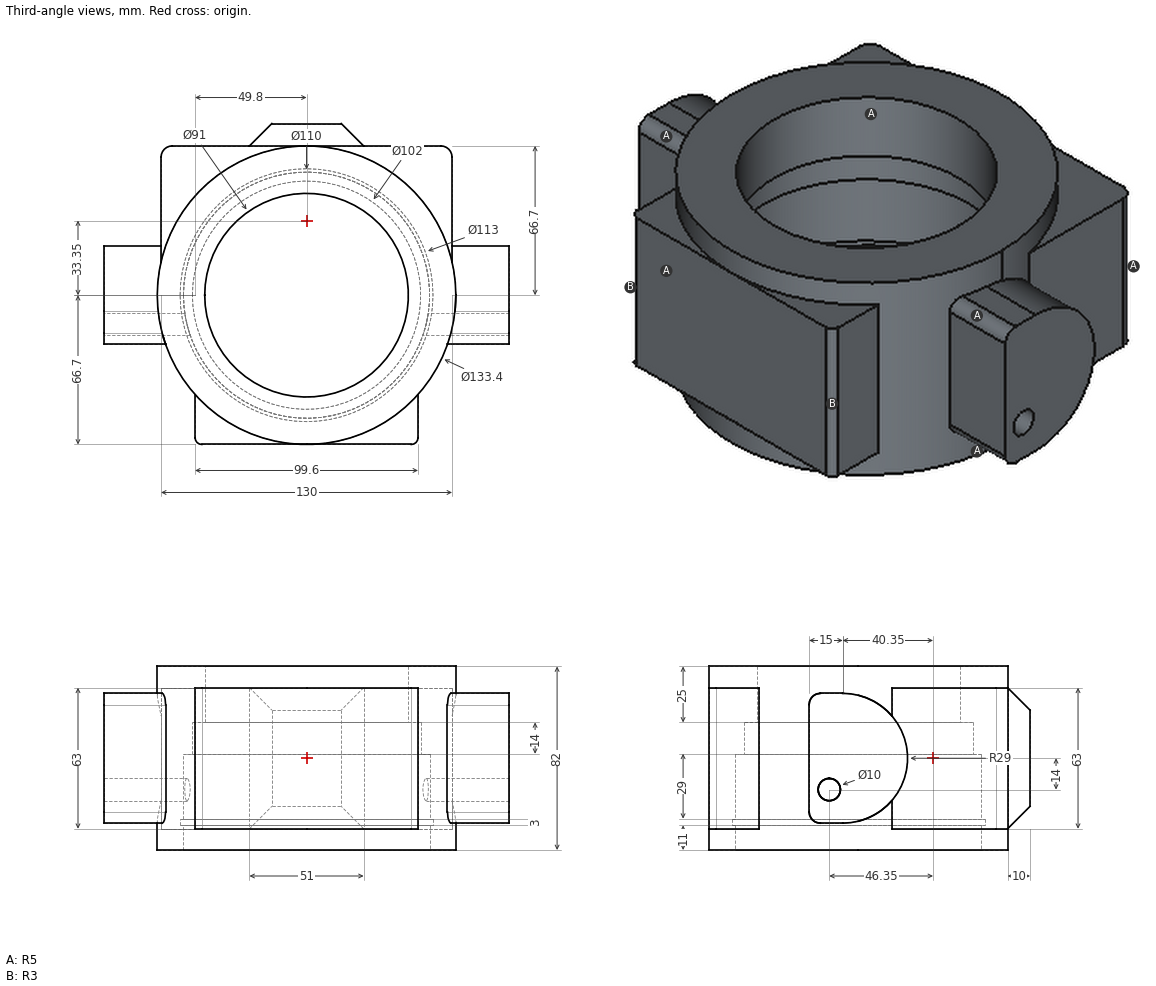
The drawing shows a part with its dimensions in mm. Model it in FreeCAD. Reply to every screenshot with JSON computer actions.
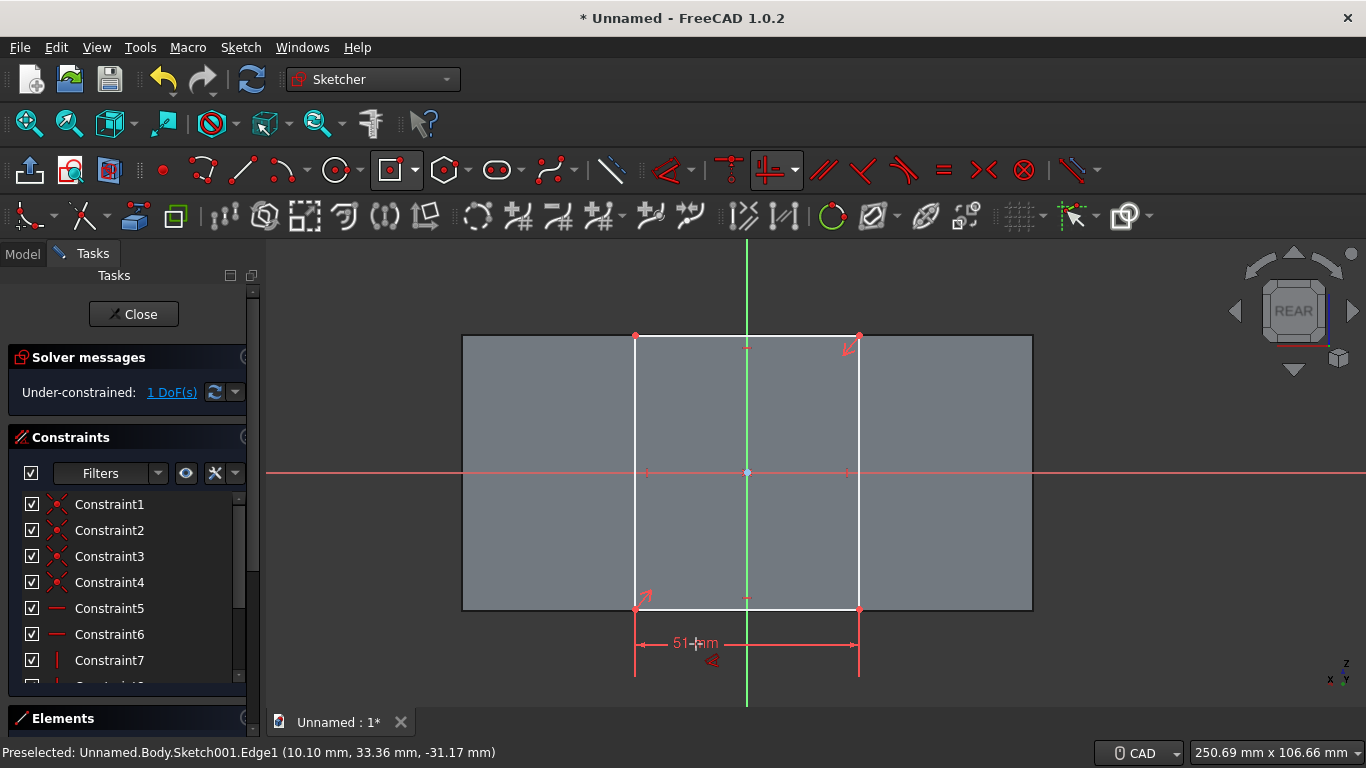
{"action": "left_click", "coordinate": [859, 527]}
{"action": "left_click", "coordinate": [893, 410]}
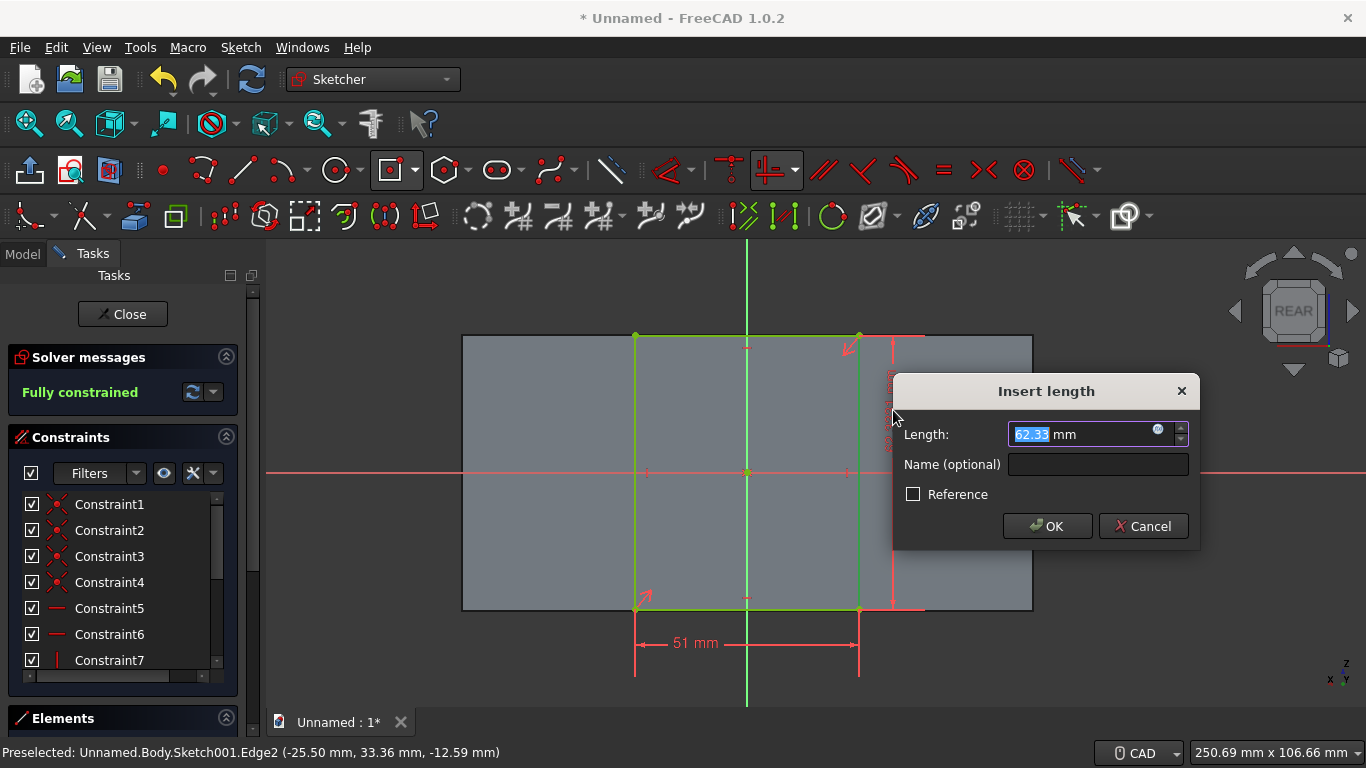
{"action": "type", "text": "63"}
{"action": "key", "text": "Return"}
{"action": "key", "text": "Escape"}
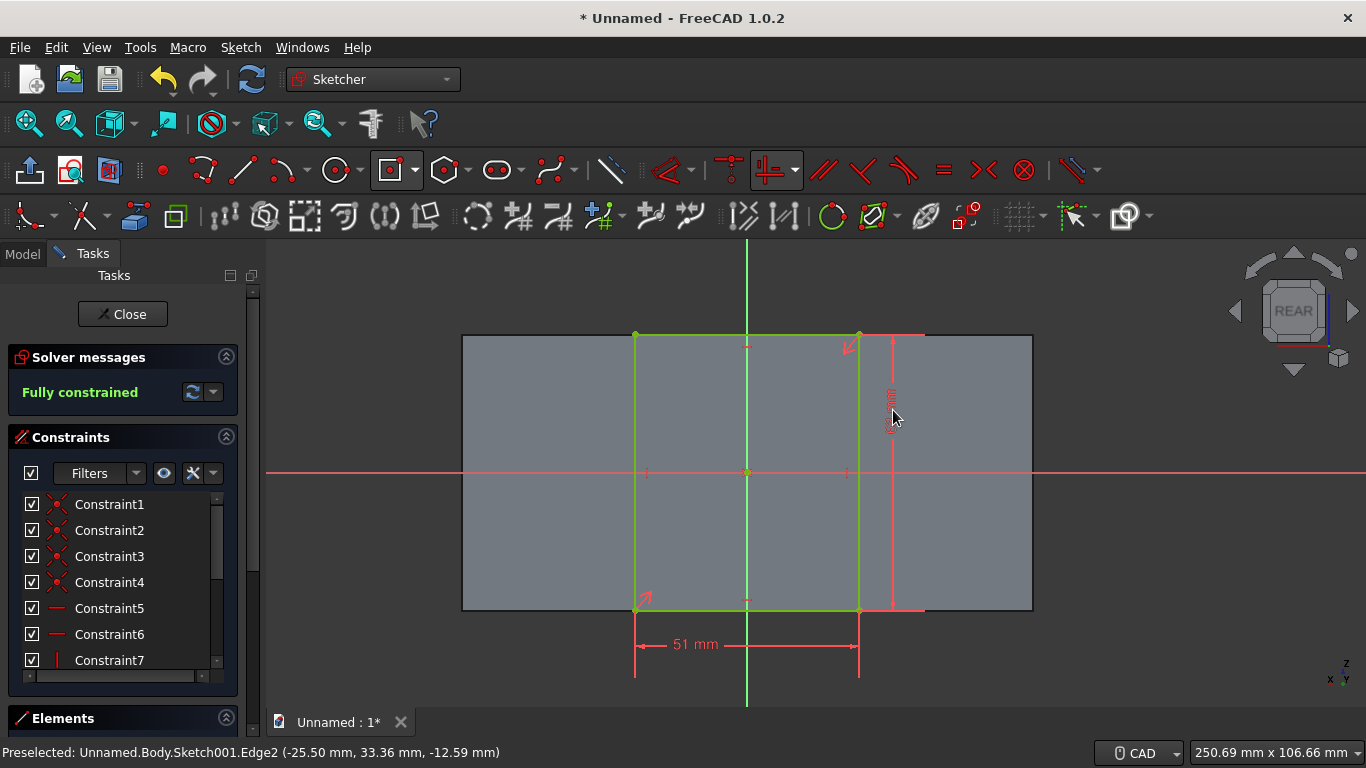
{"action": "left_click", "coordinate": [123, 314]}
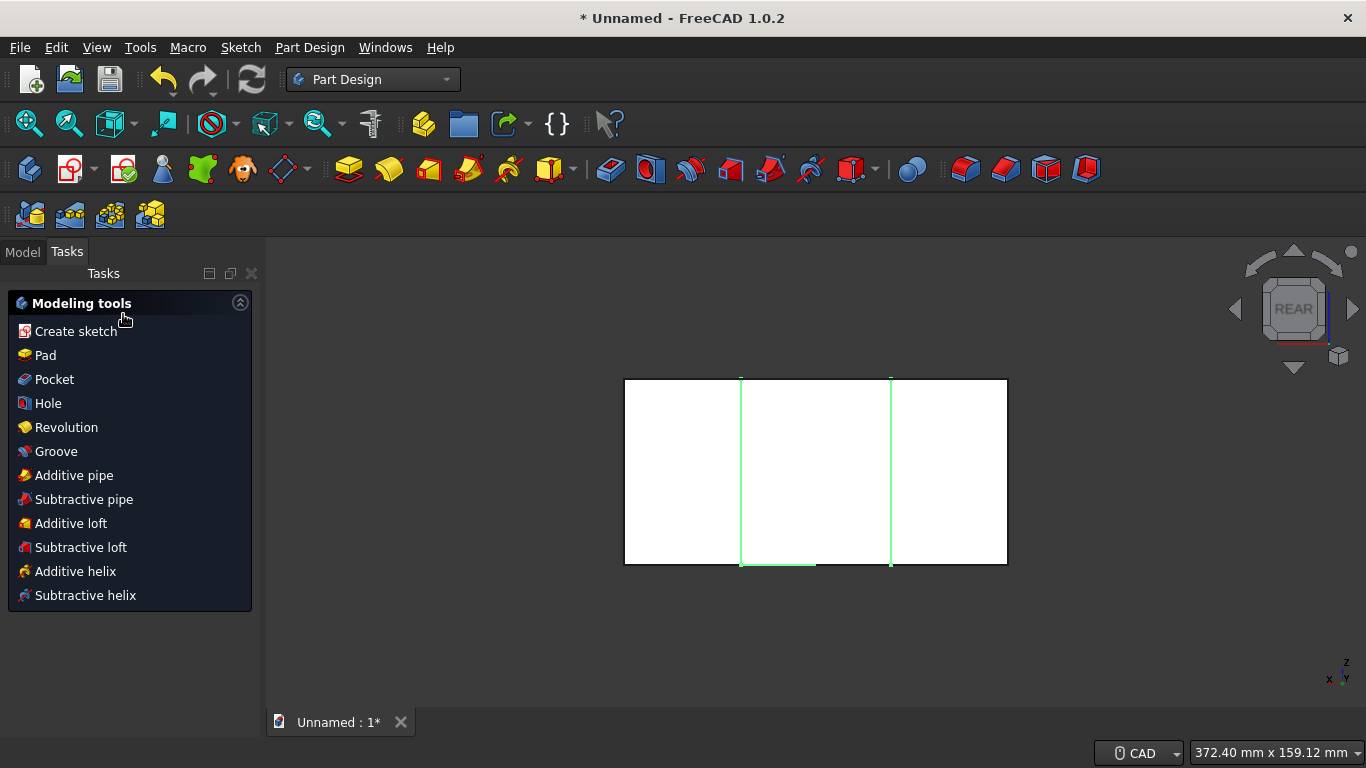
{"action": "left_click", "coordinate": [350, 170]}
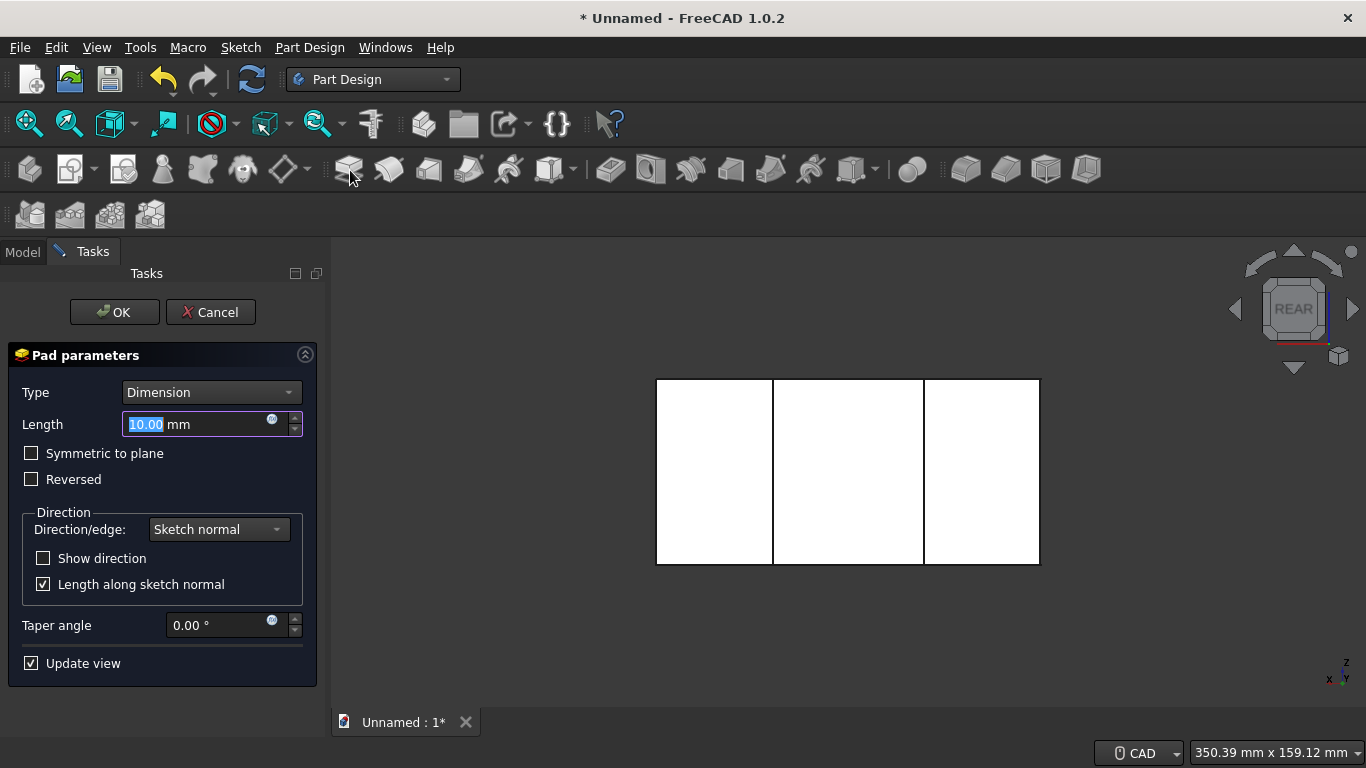
{"action": "type", "text": "10"}
{"action": "key", "text": "Tab"}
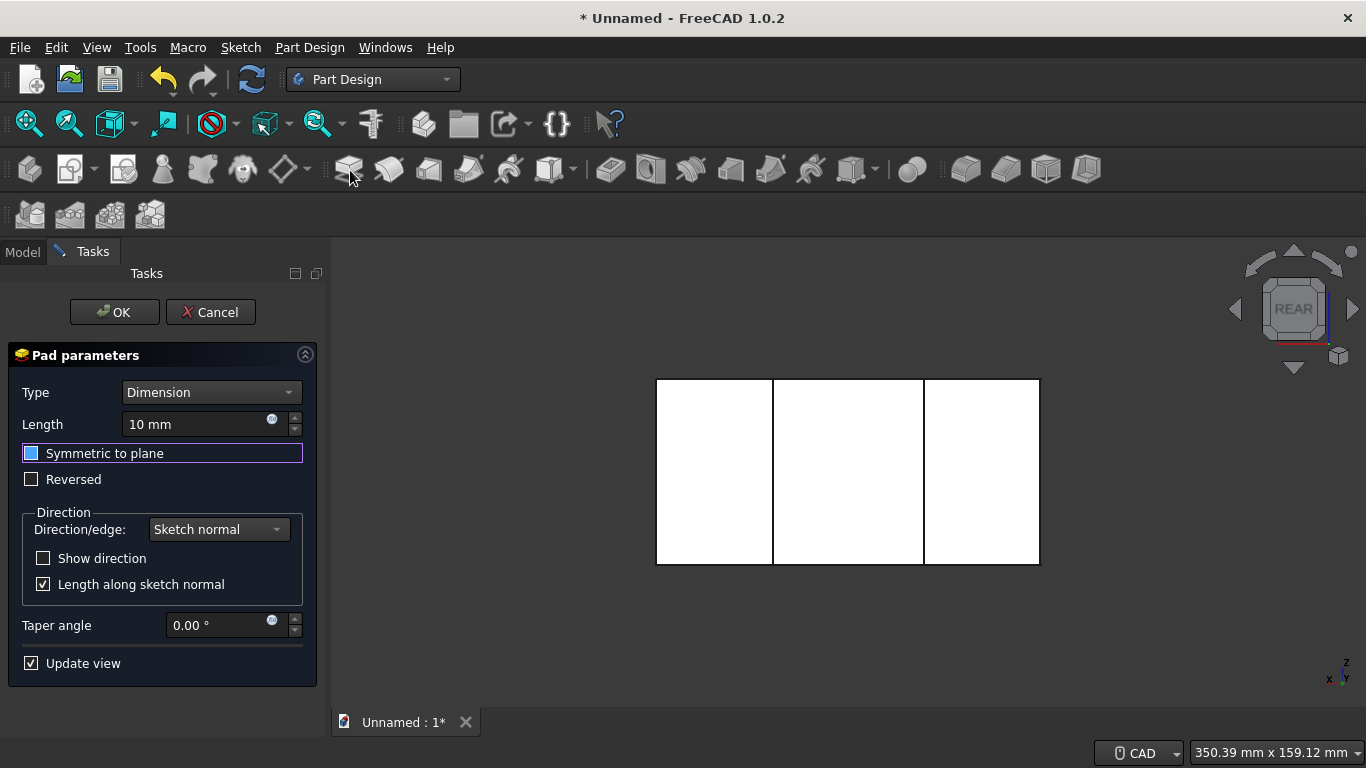
{"action": "triple_click", "coordinate": [226, 625]}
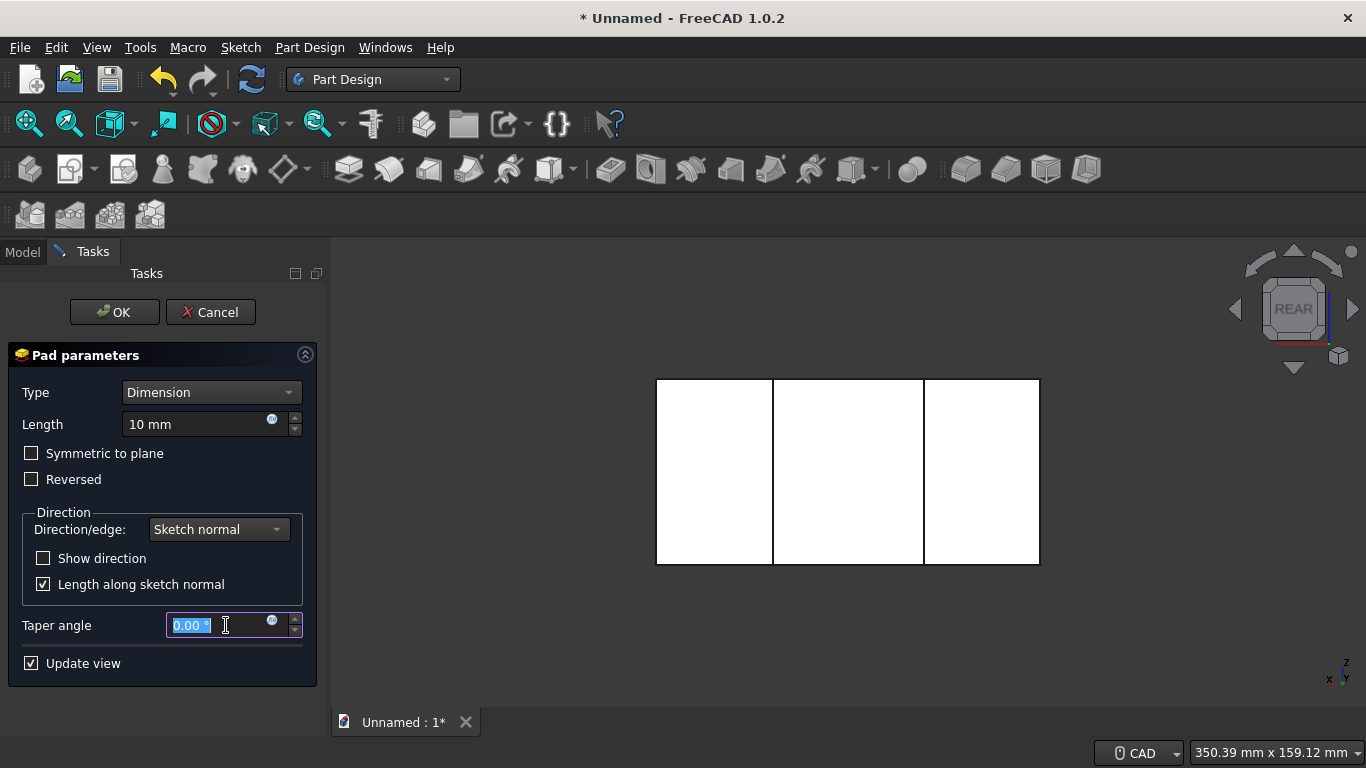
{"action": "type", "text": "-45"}
{"action": "key", "text": "Tab"}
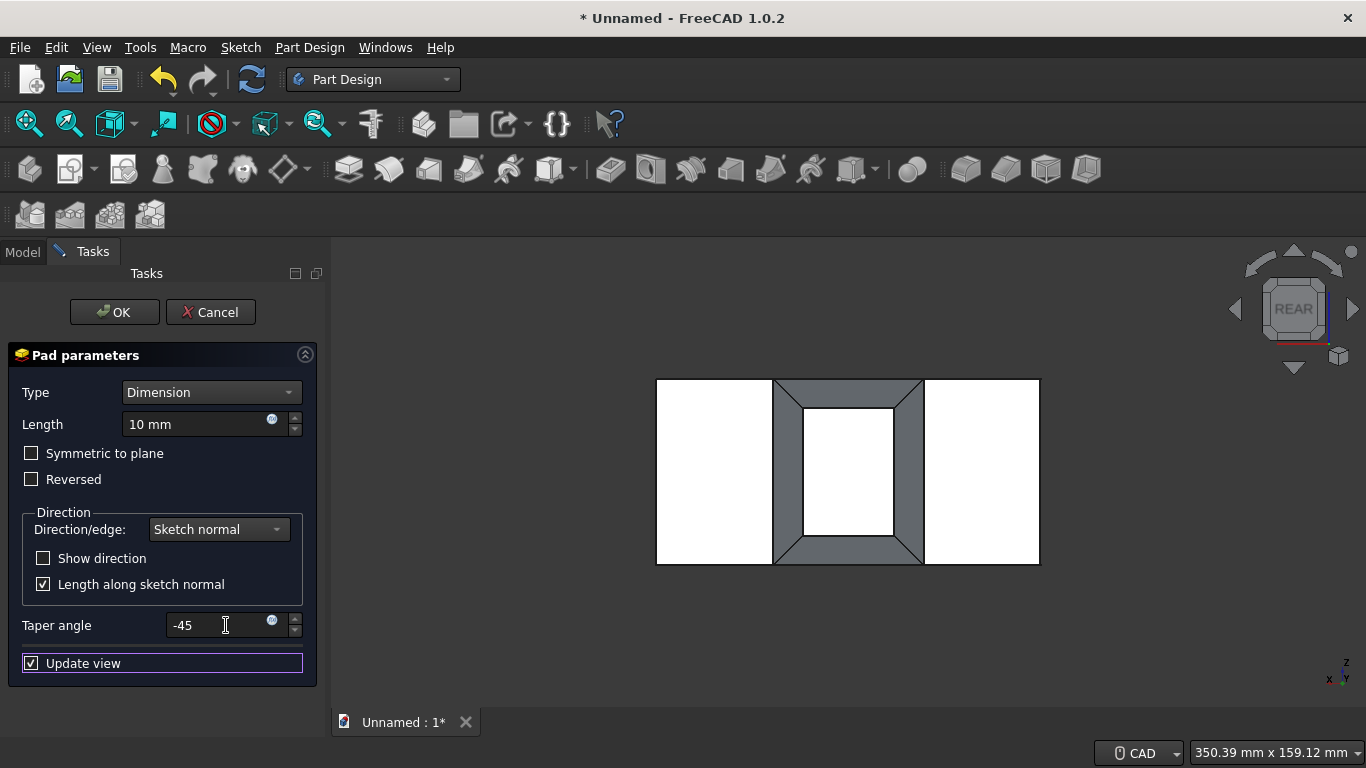
{"action": "left_click", "coordinate": [115, 312]}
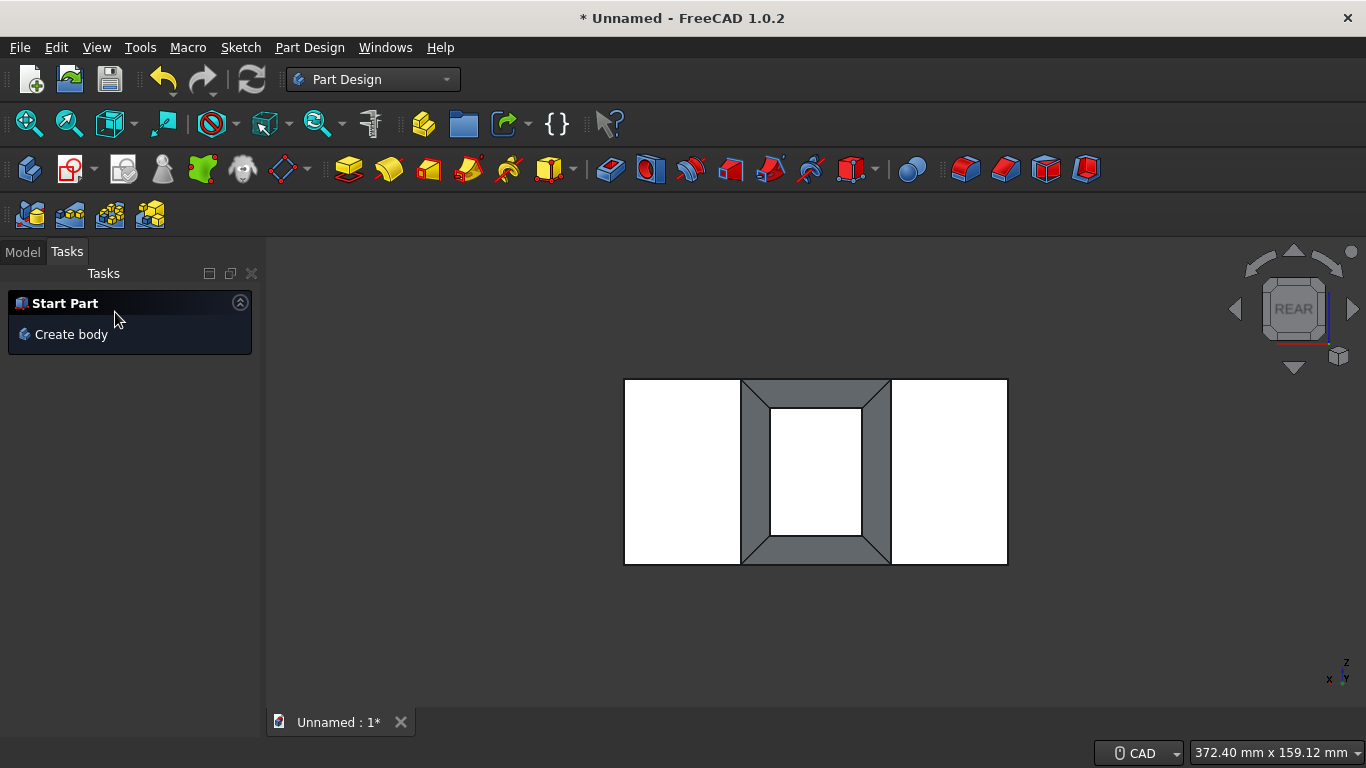
{"action": "key", "text": "v f"}